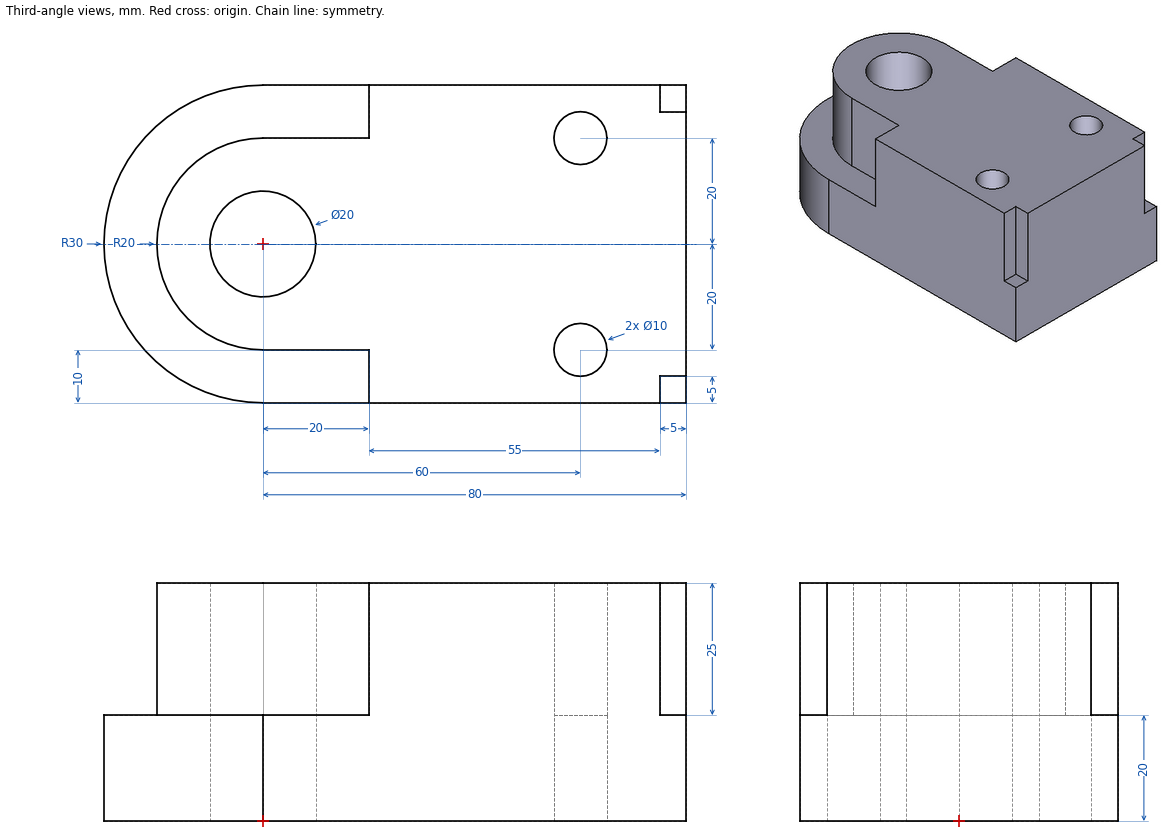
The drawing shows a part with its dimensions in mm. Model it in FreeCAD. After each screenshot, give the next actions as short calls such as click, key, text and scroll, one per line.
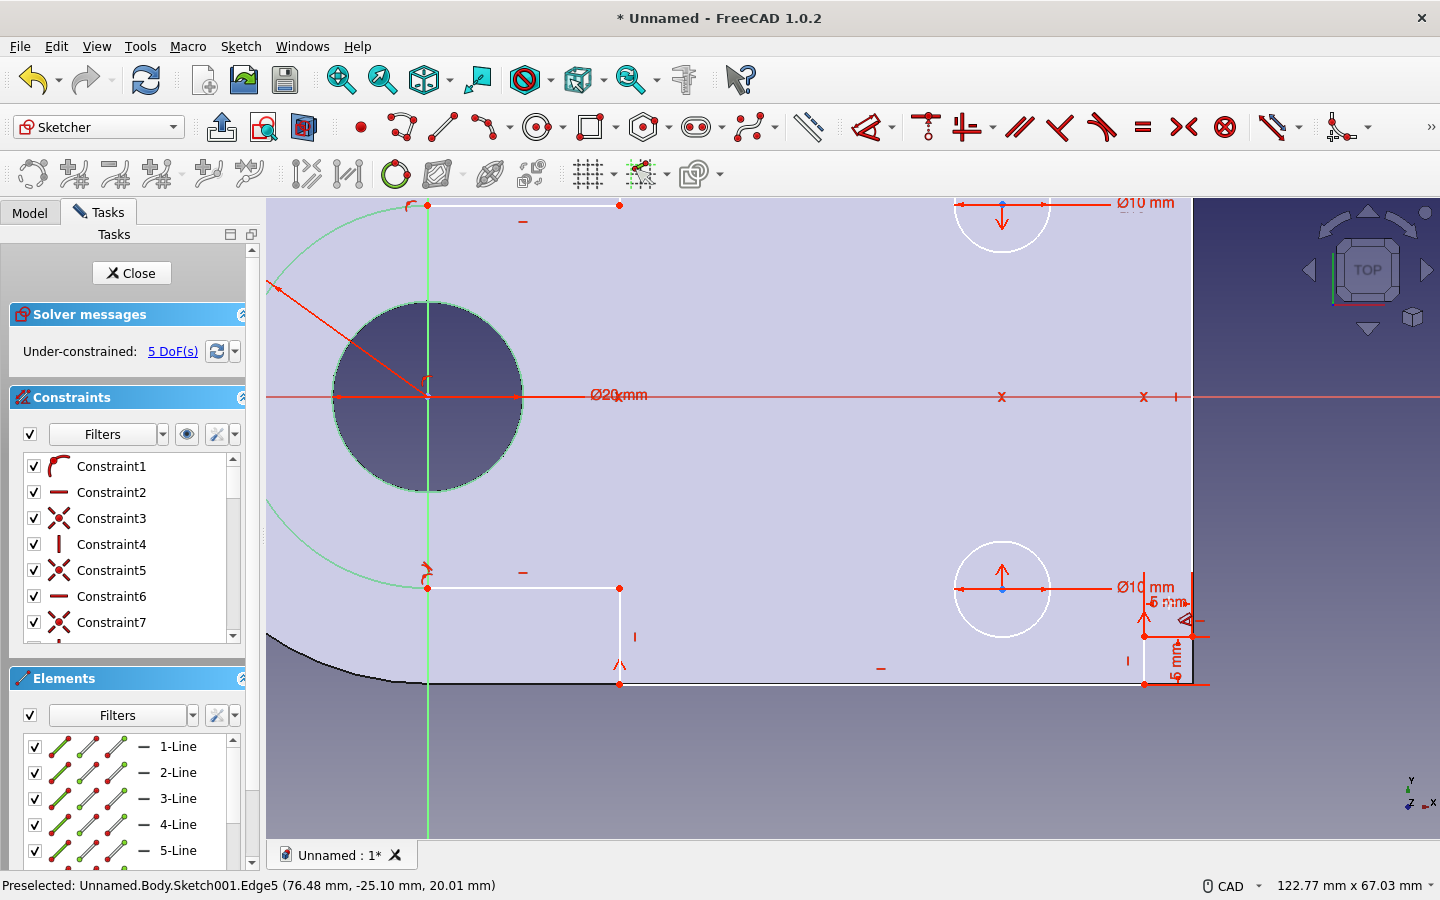
click(485, 588)
click(524, 622)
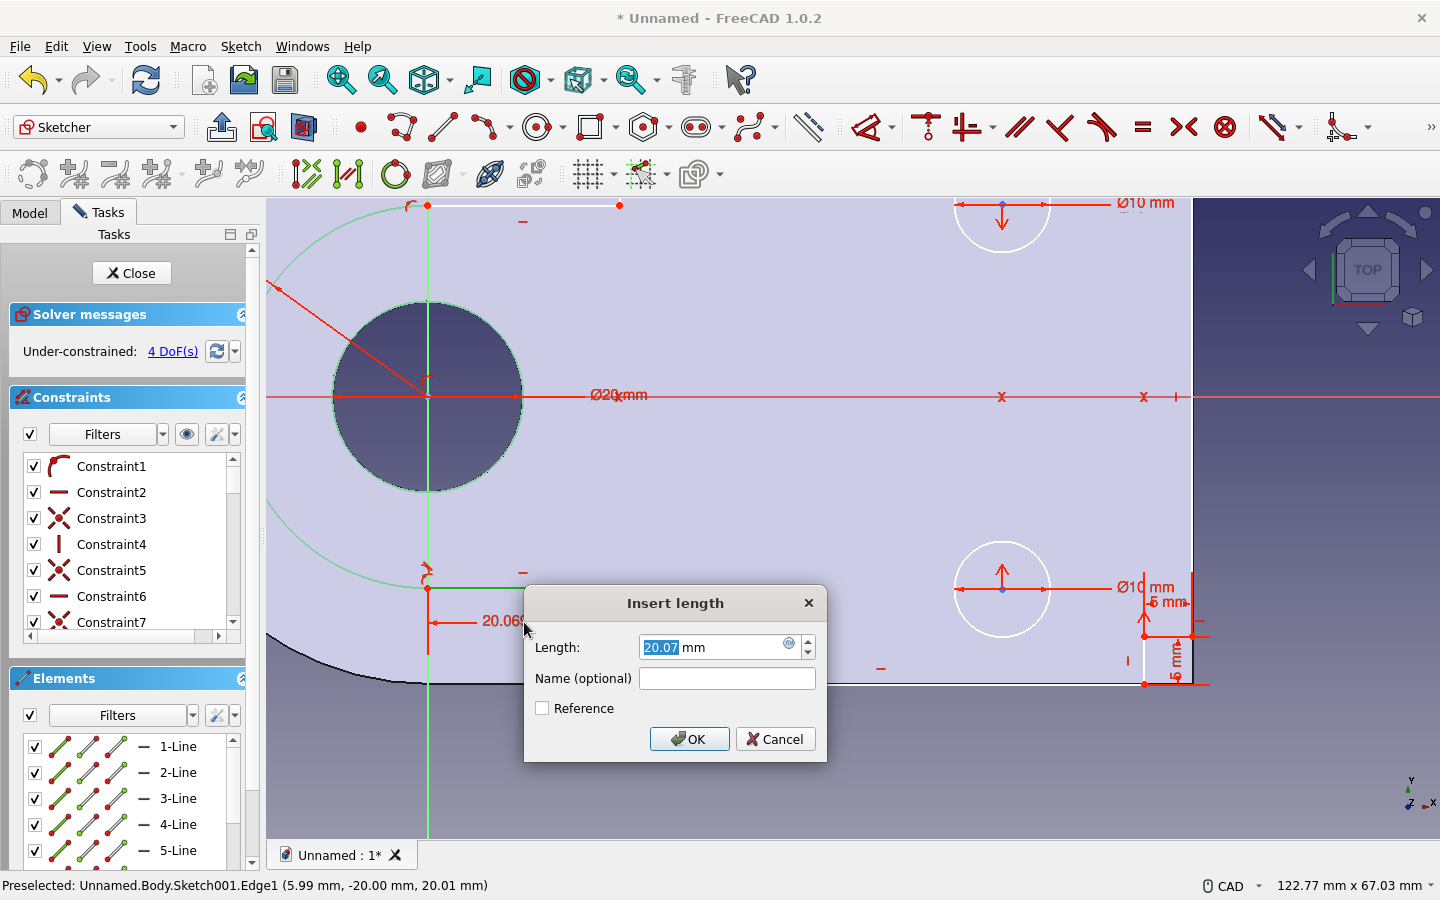
text(20)
key(Return)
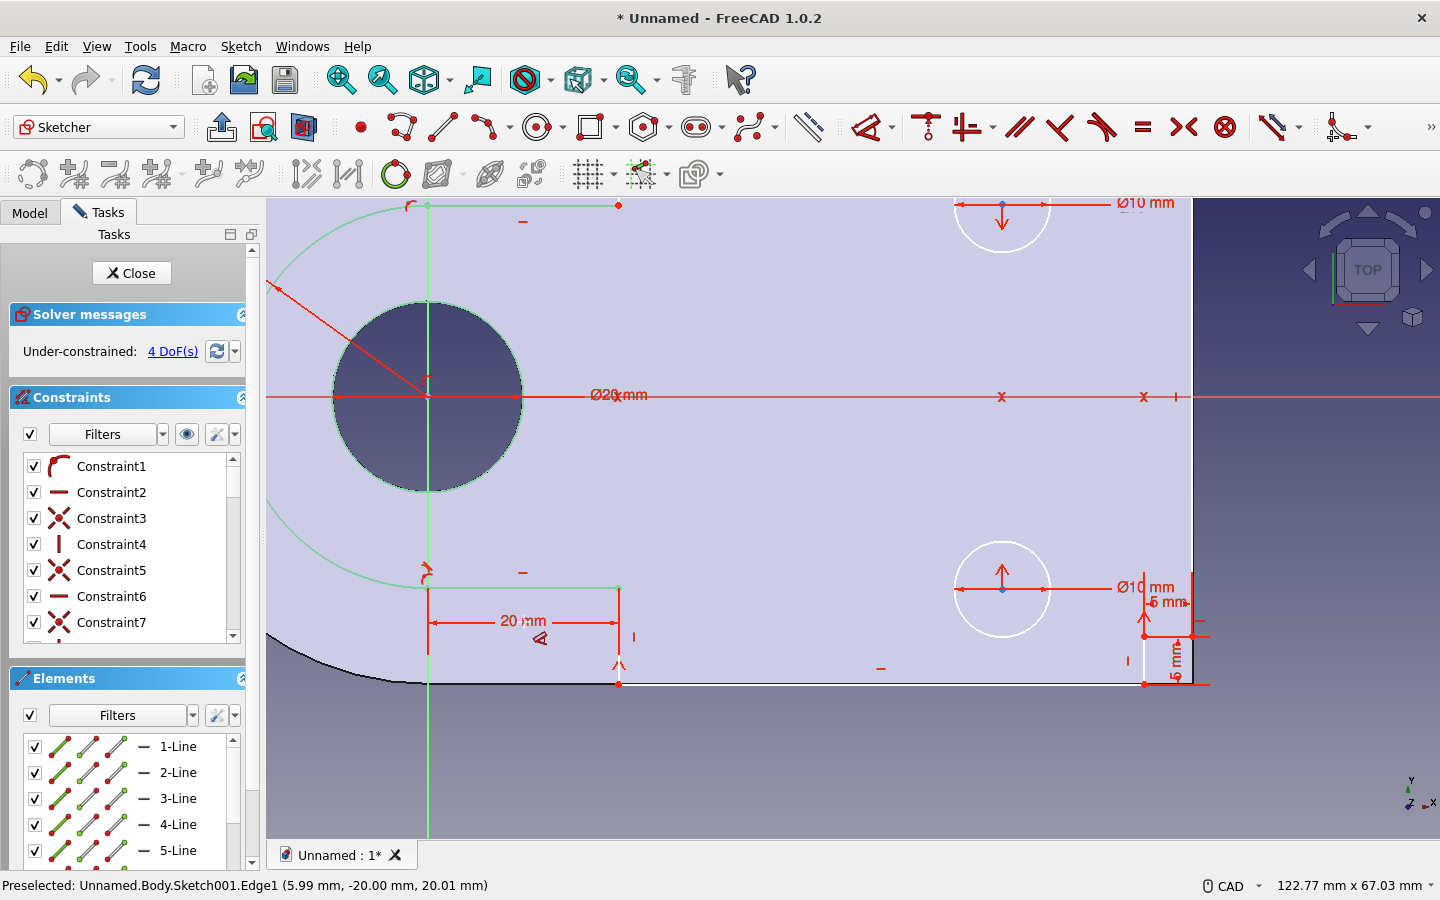
click(619, 617)
click(585, 659)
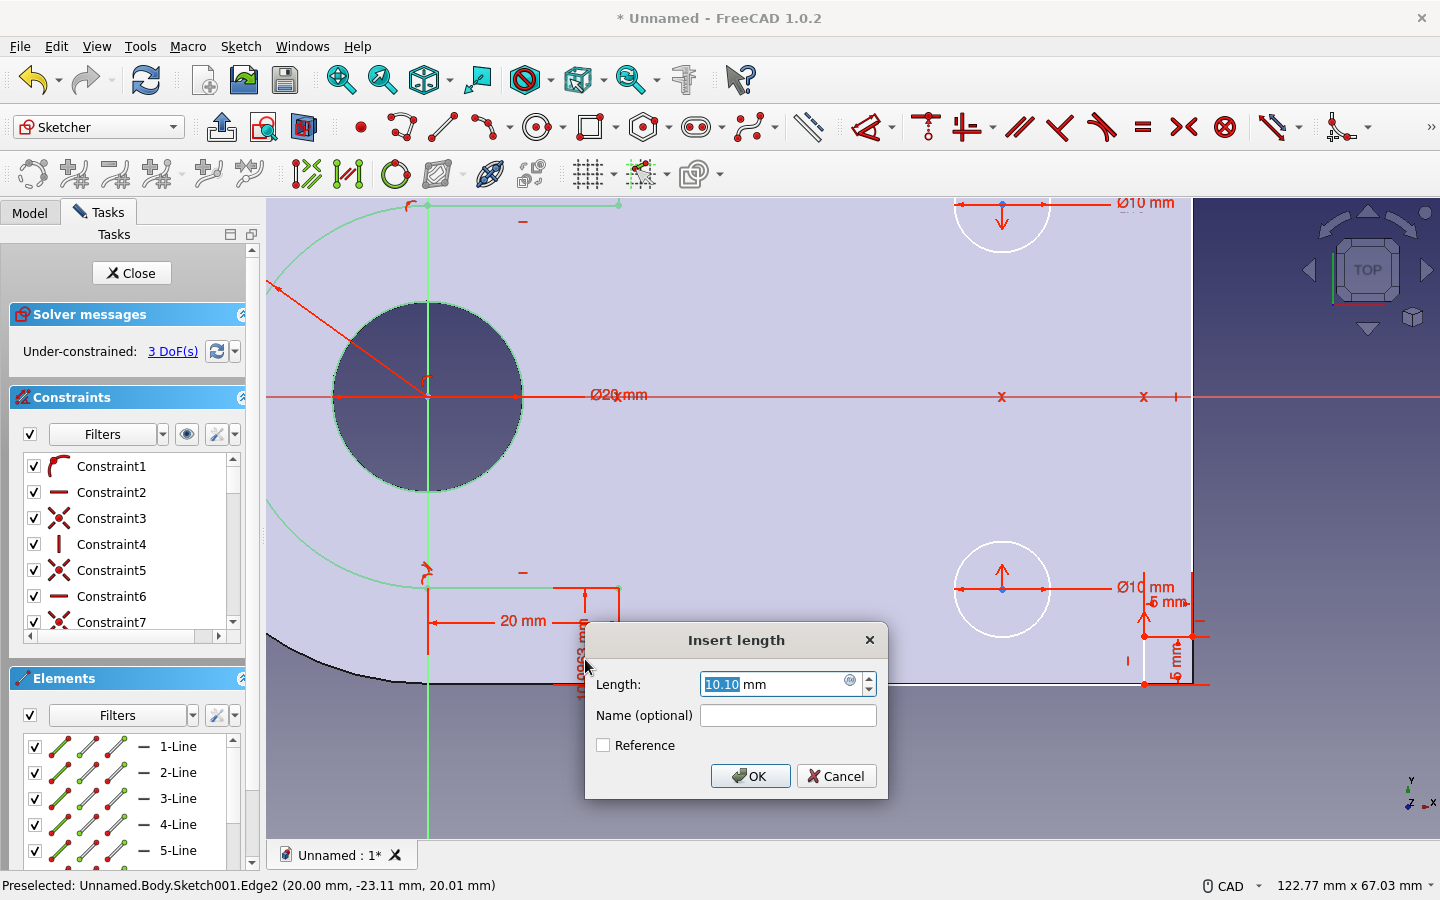
text(10)
key(Return)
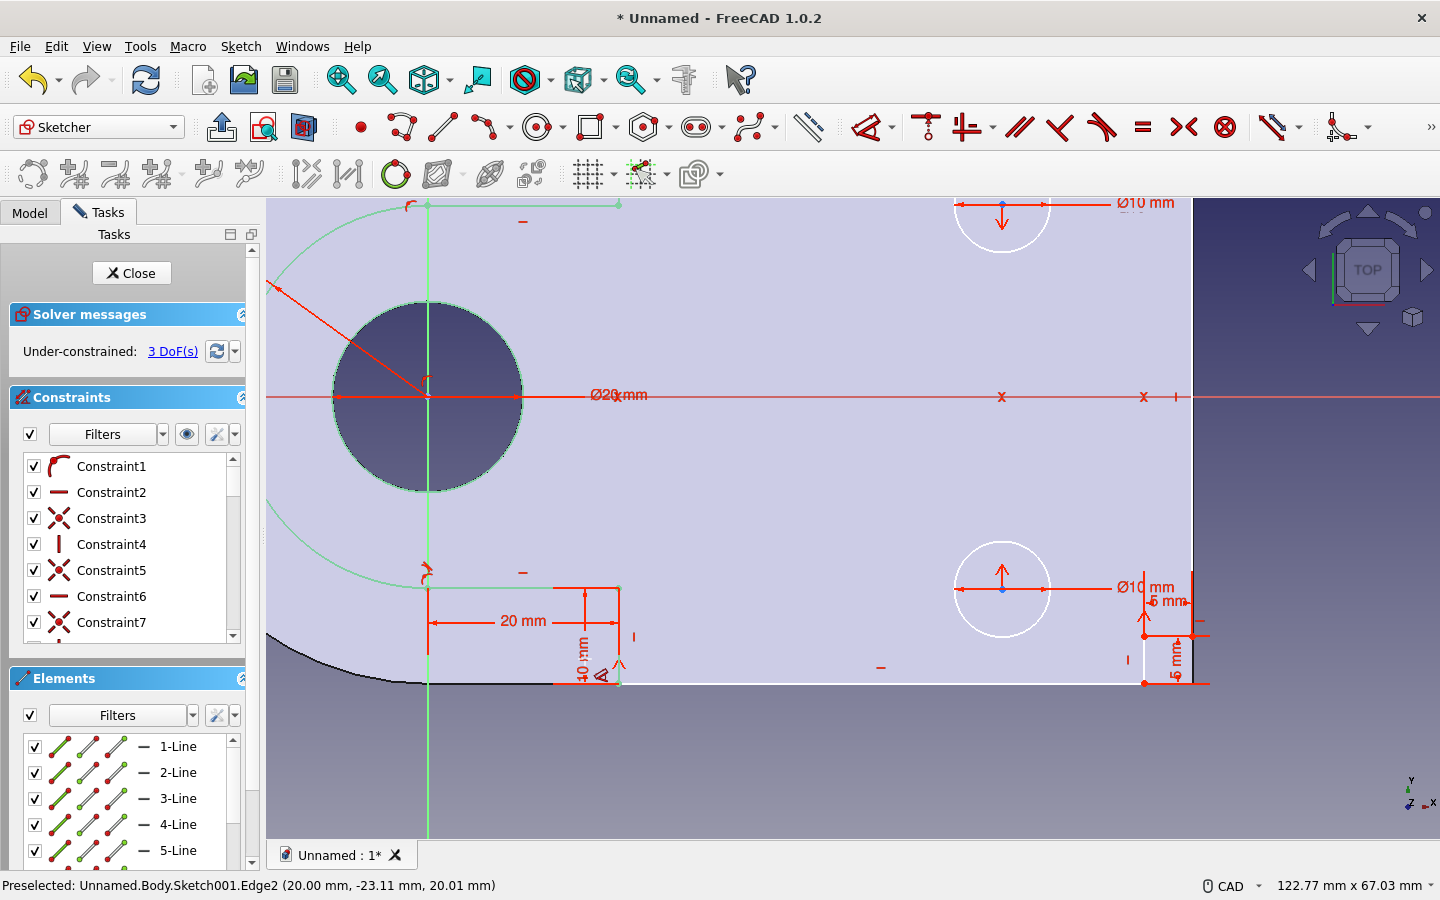
click(777, 684)
click(882, 718)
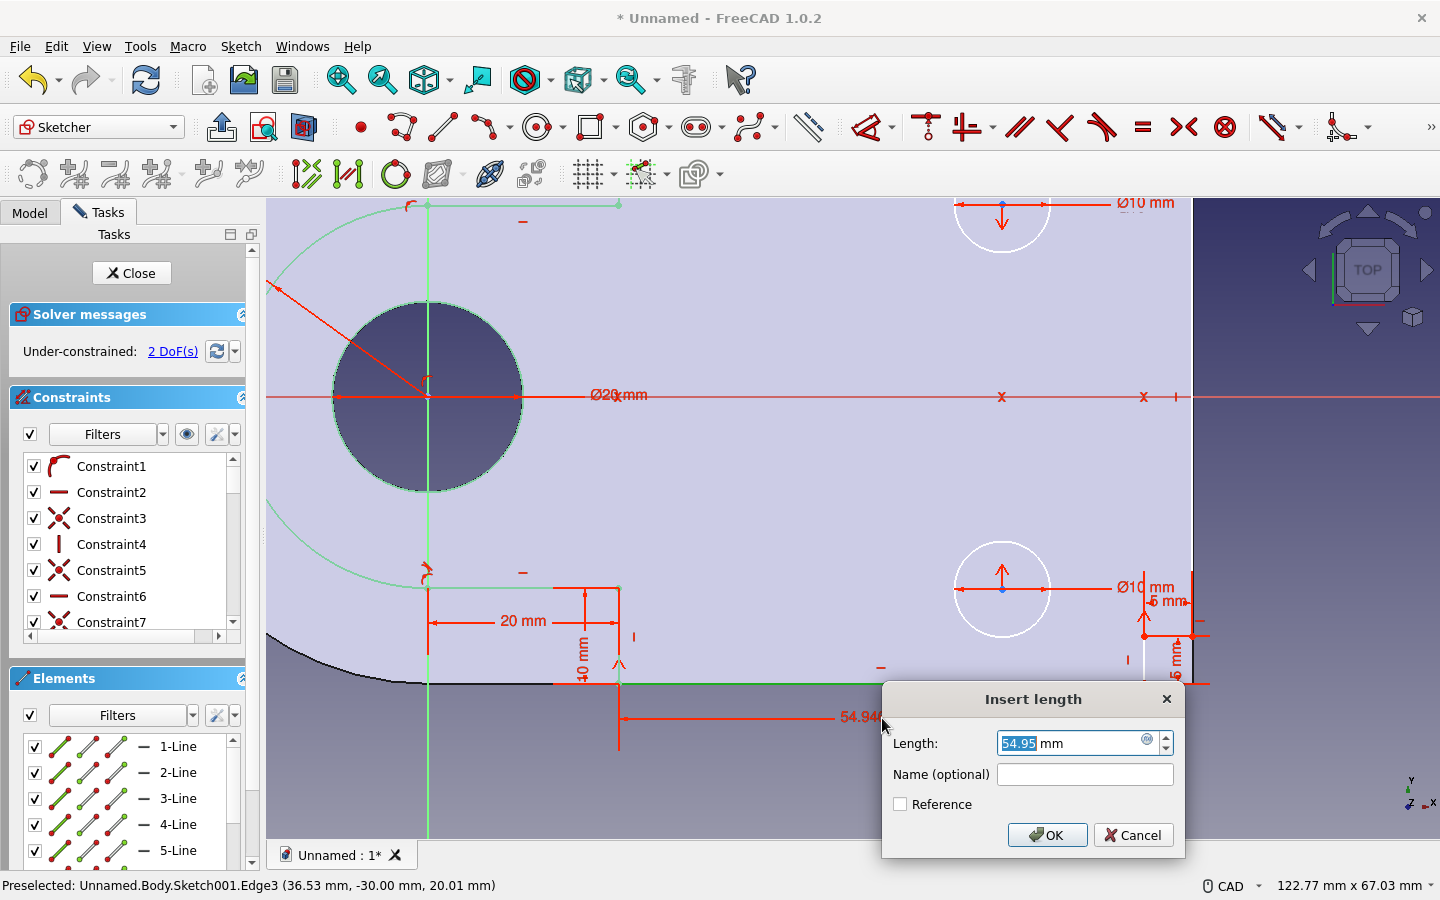
text(55)
key(Return)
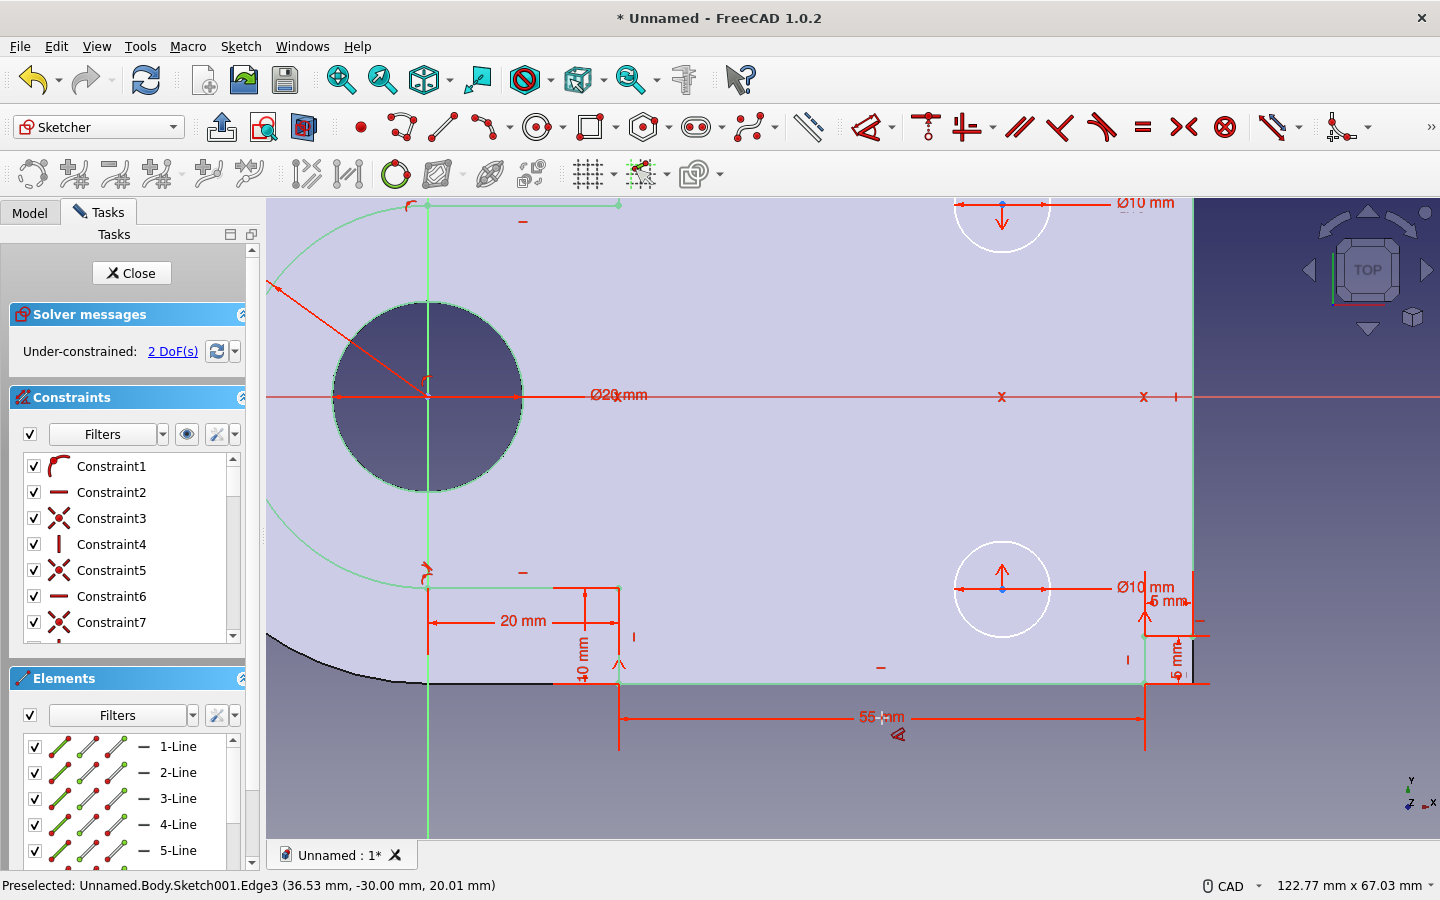
click(1002, 589)
click(715, 623)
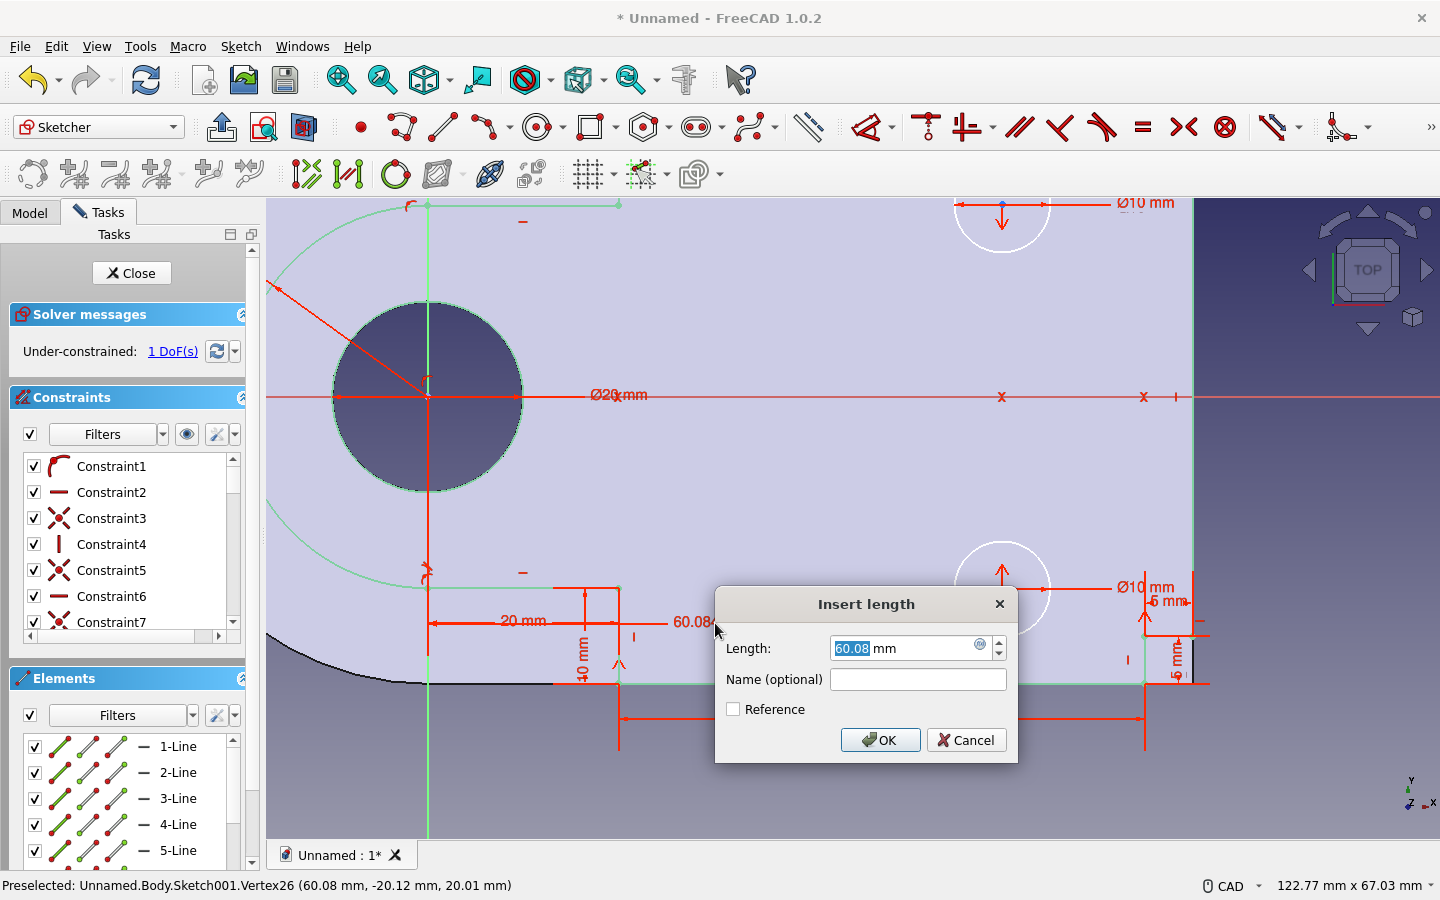
text(60)
key(Return)